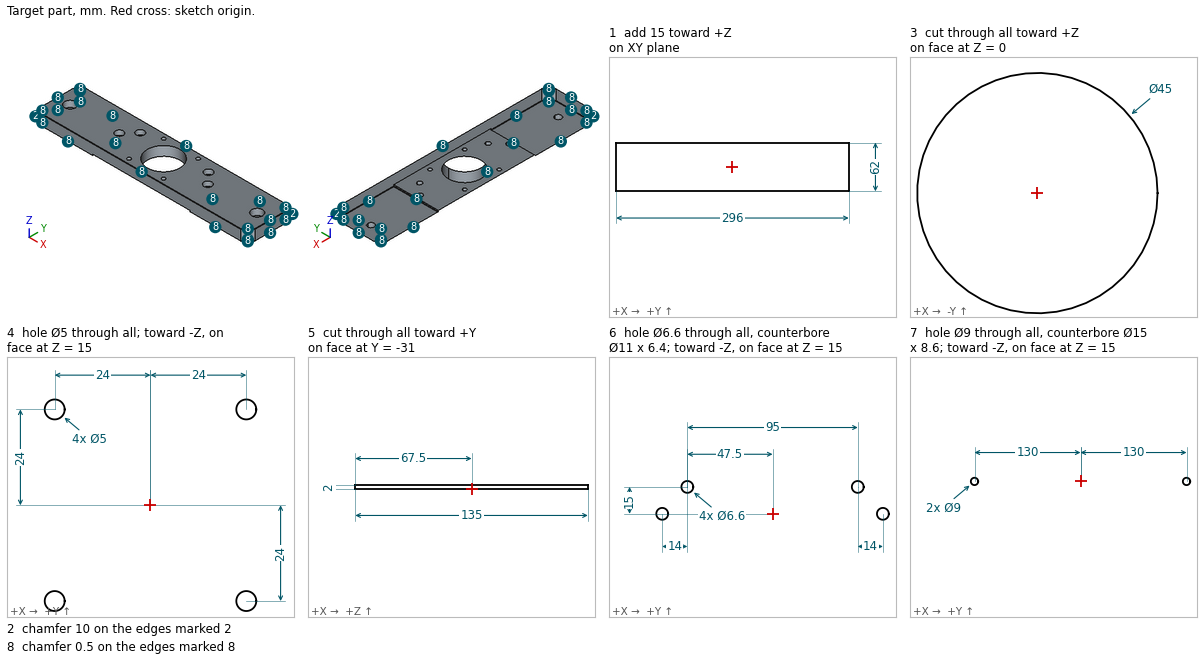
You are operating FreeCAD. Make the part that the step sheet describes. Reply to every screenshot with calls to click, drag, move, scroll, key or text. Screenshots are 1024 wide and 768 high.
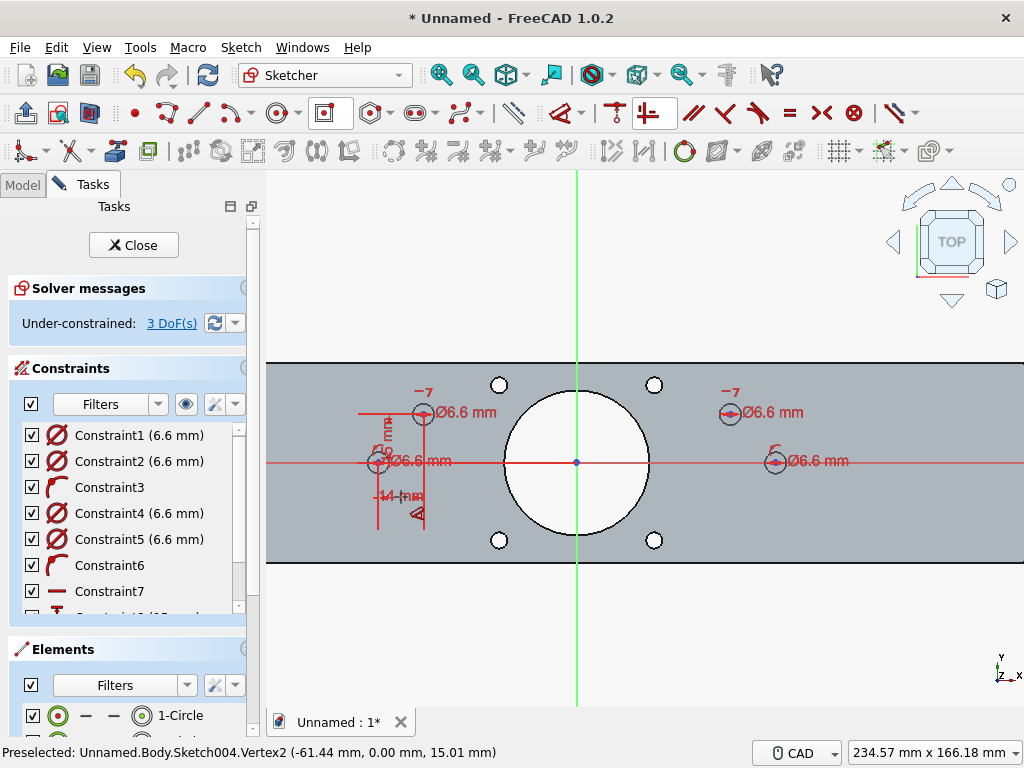
click(424, 414)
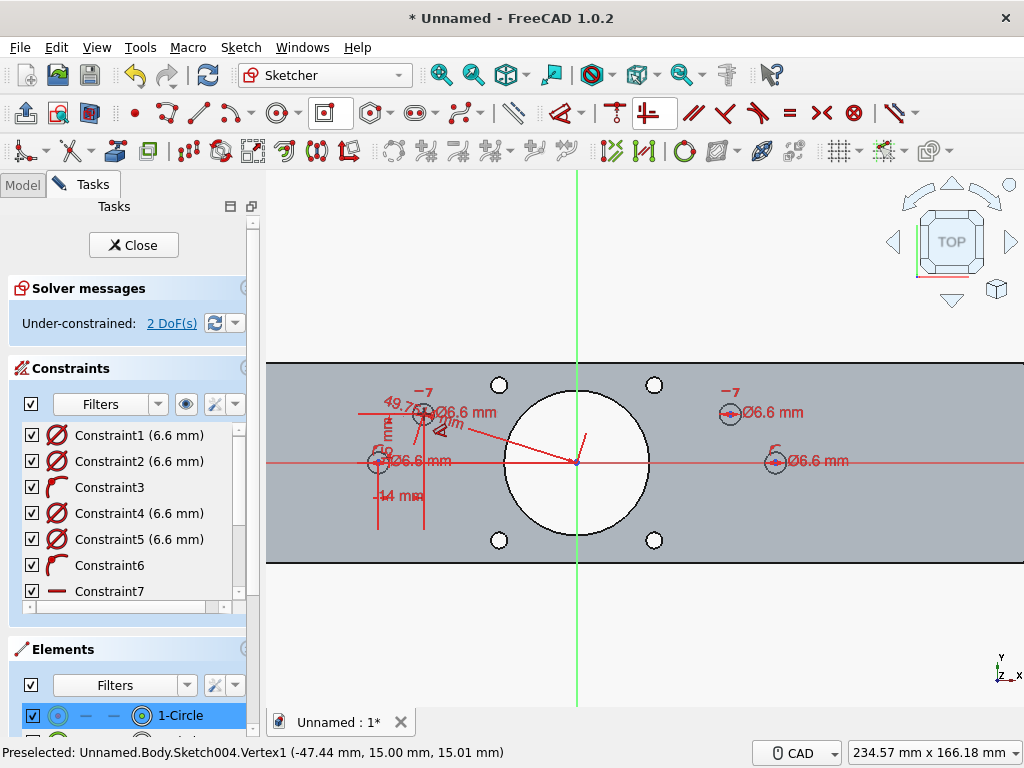
click(730, 414)
click(506, 380)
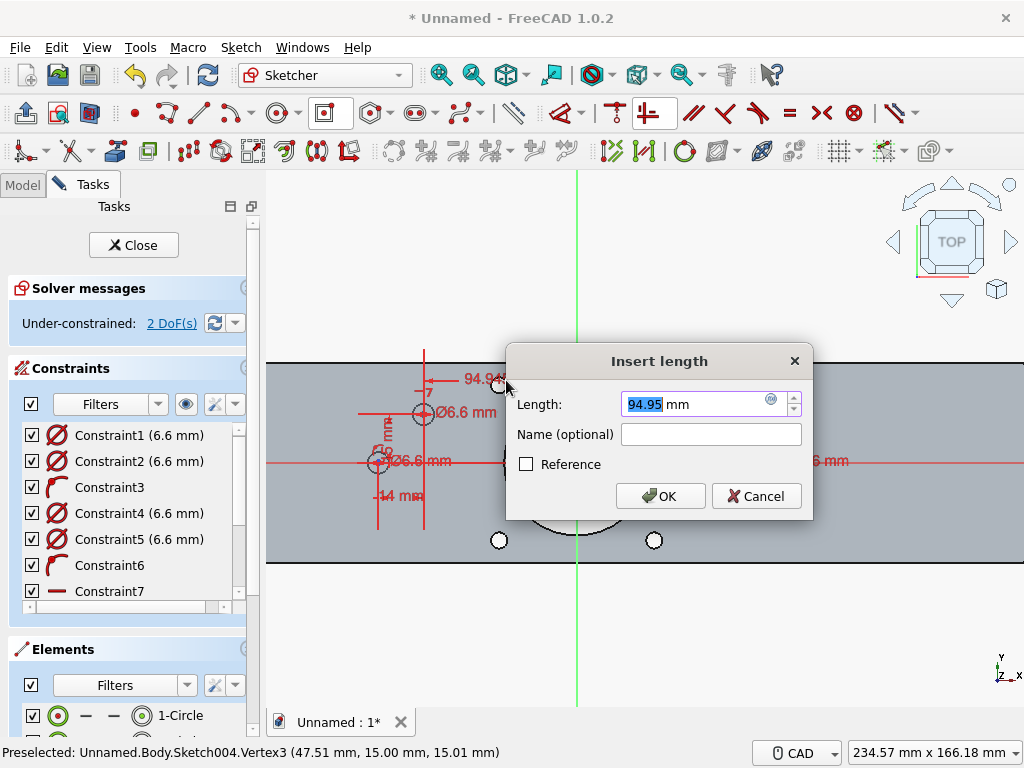
text(95)
key(Return)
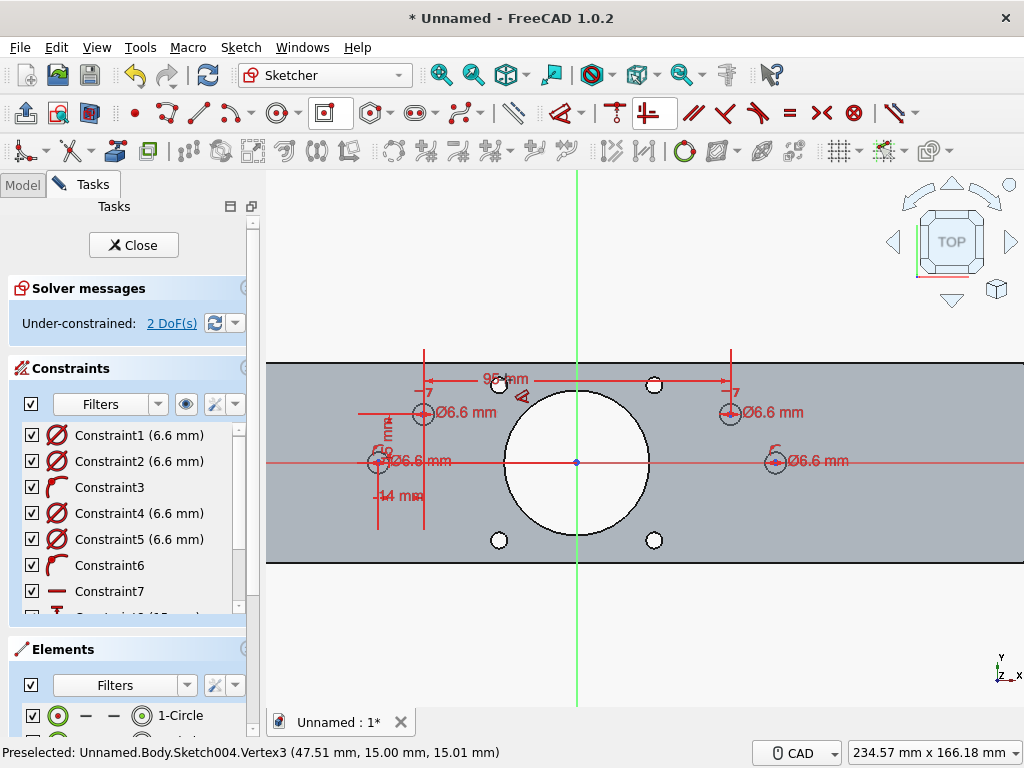
click(731, 414)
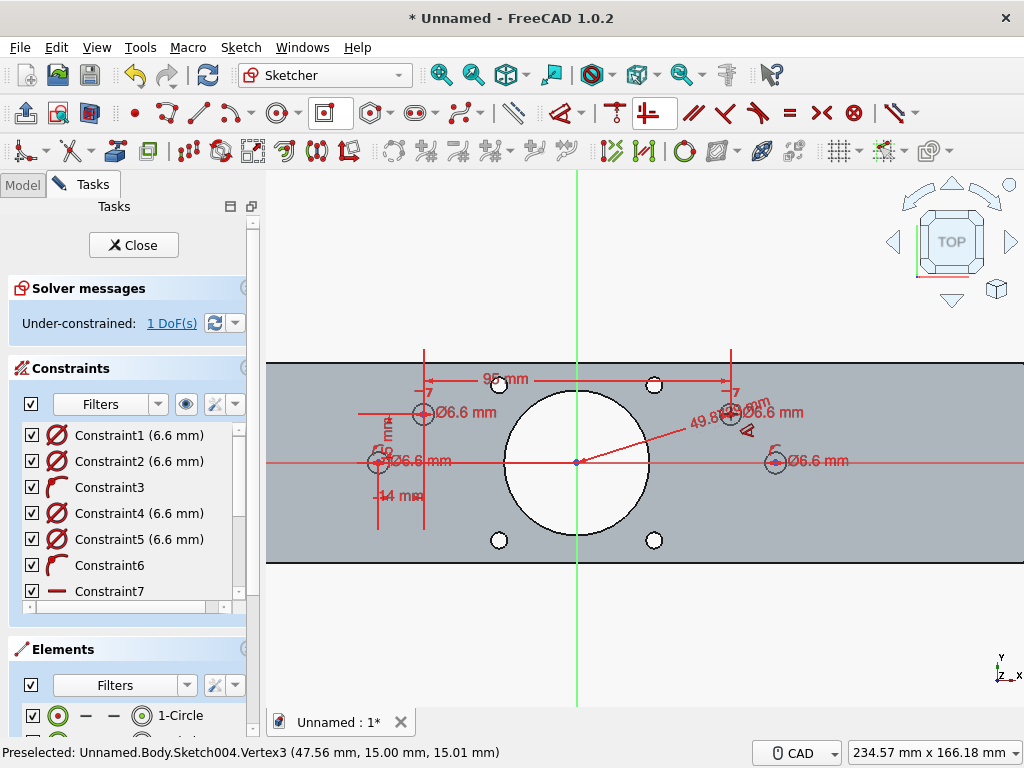
click(776, 463)
click(753, 497)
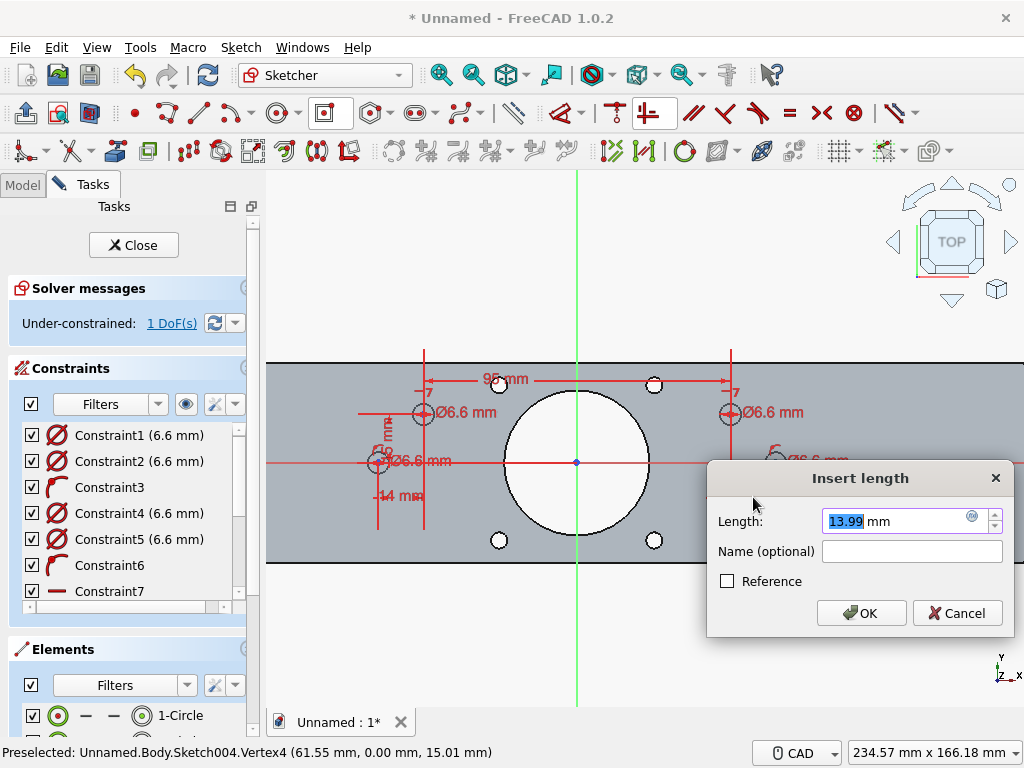
text(14)
key(Return)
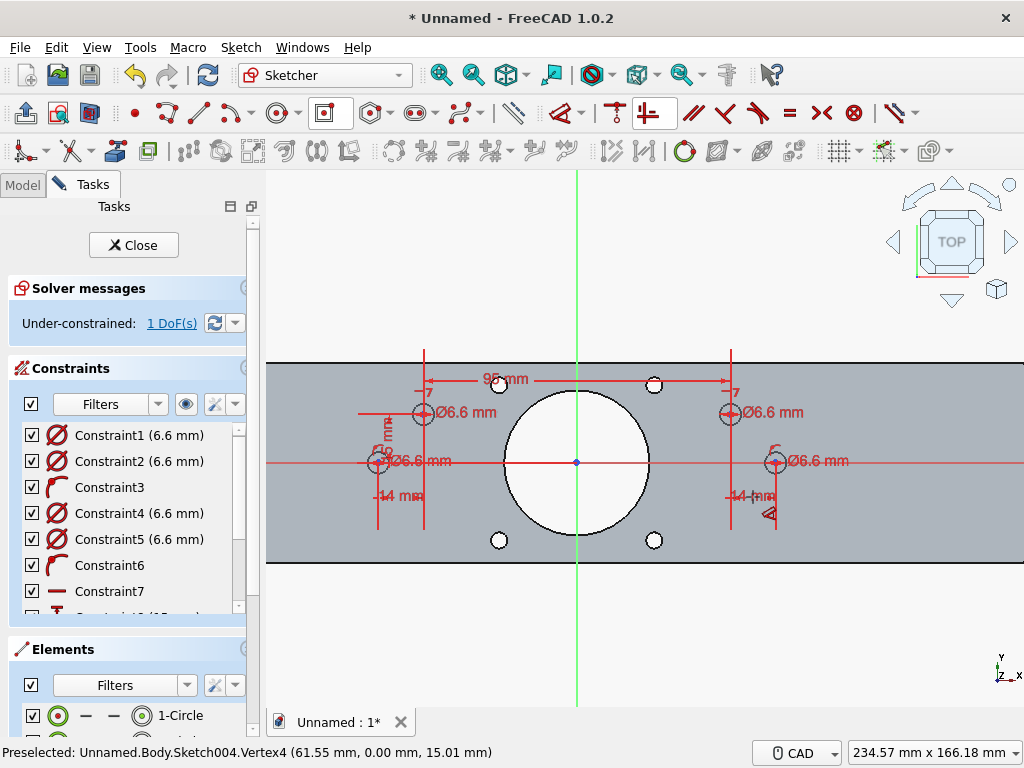
click(424, 414)
click(500, 497)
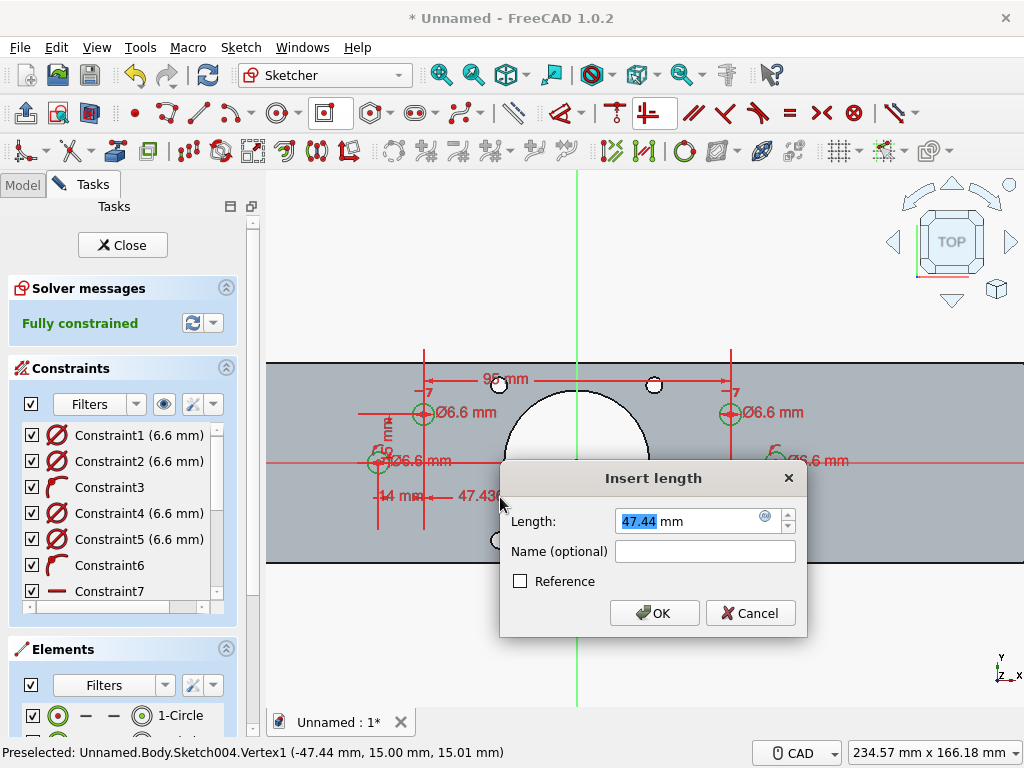
text(47.5)
key(Return)
key(Escape)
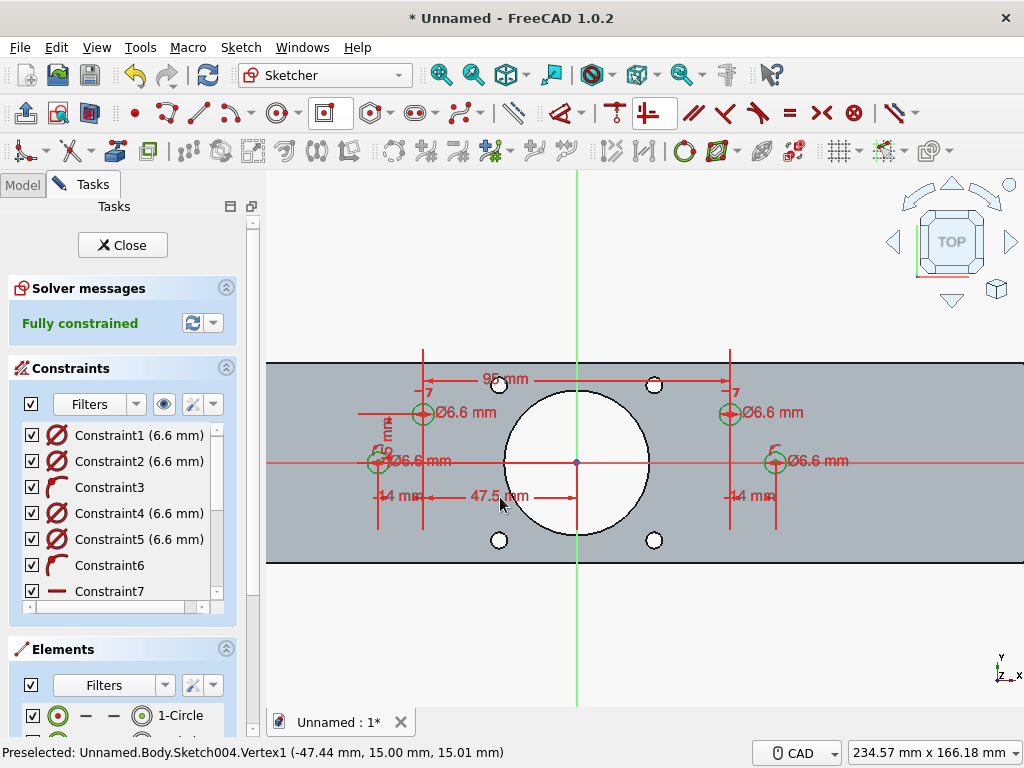
click(123, 245)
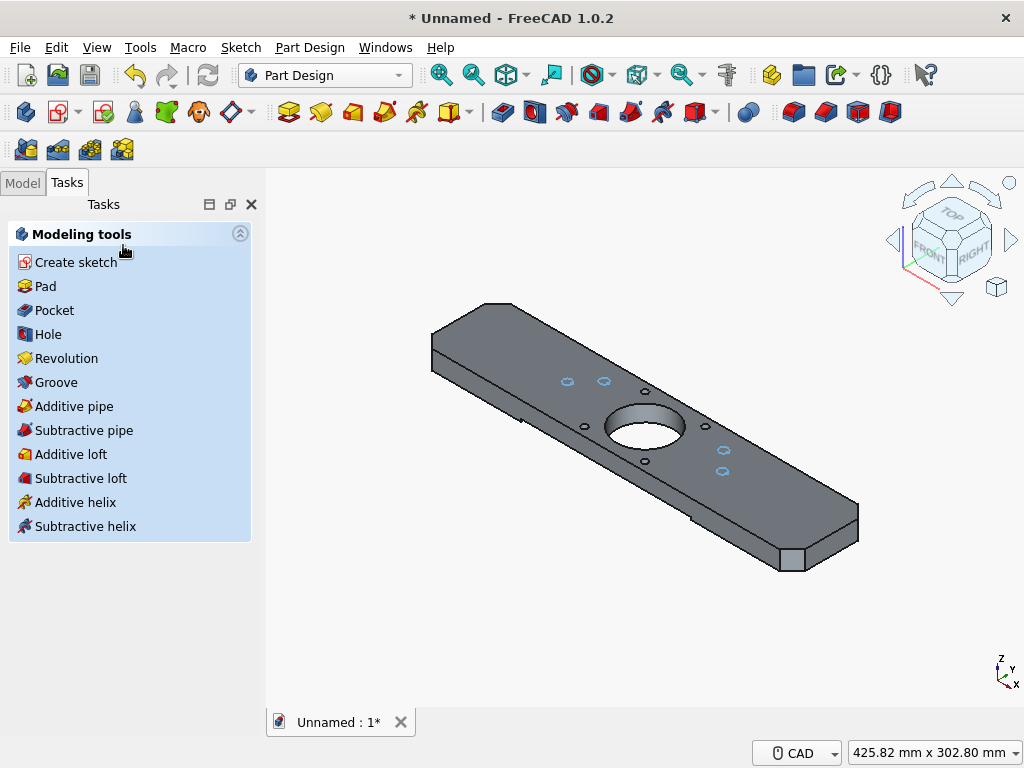
click(536, 112)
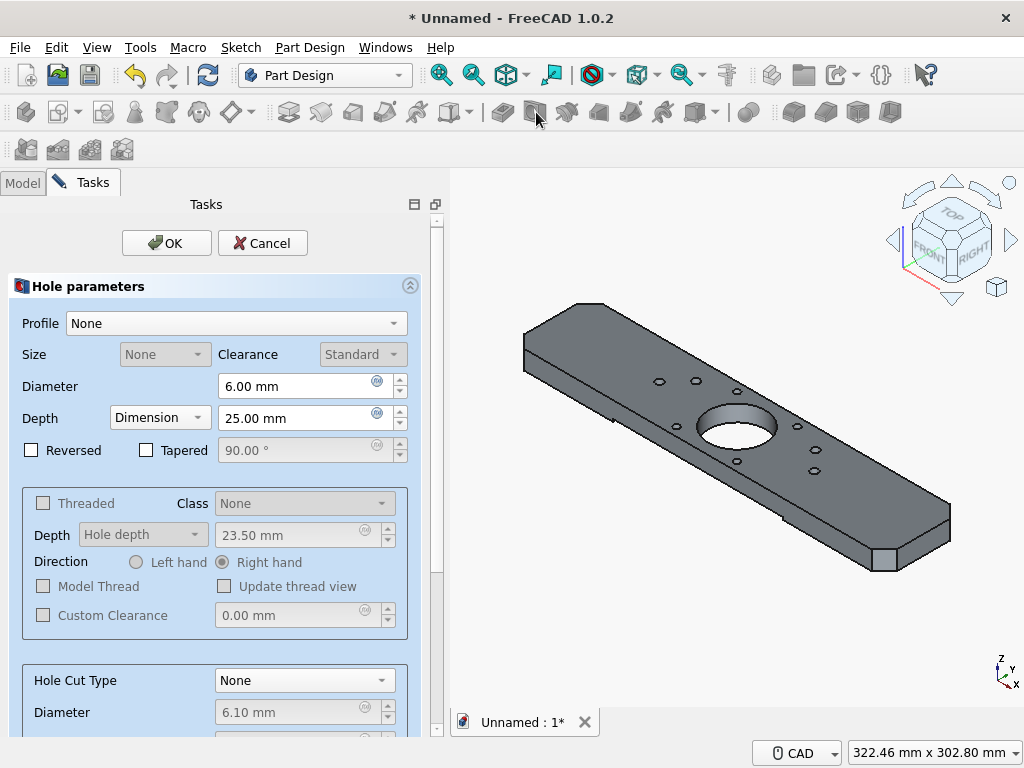
triple_click(305, 386)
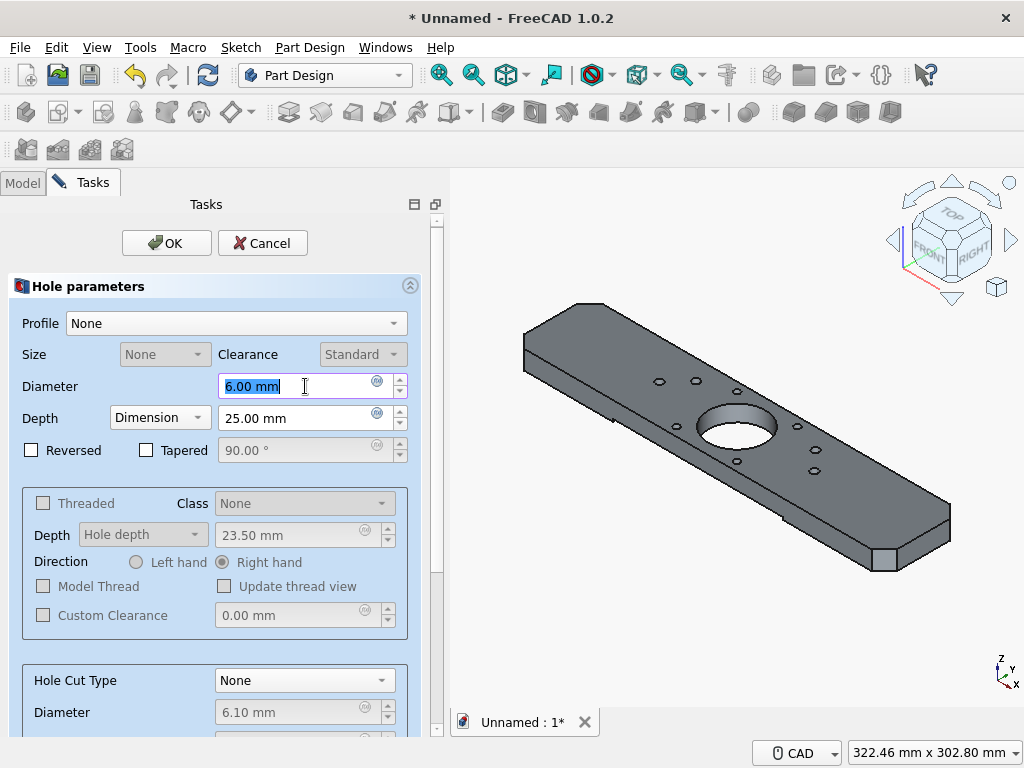
text(6.6)
key(Tab)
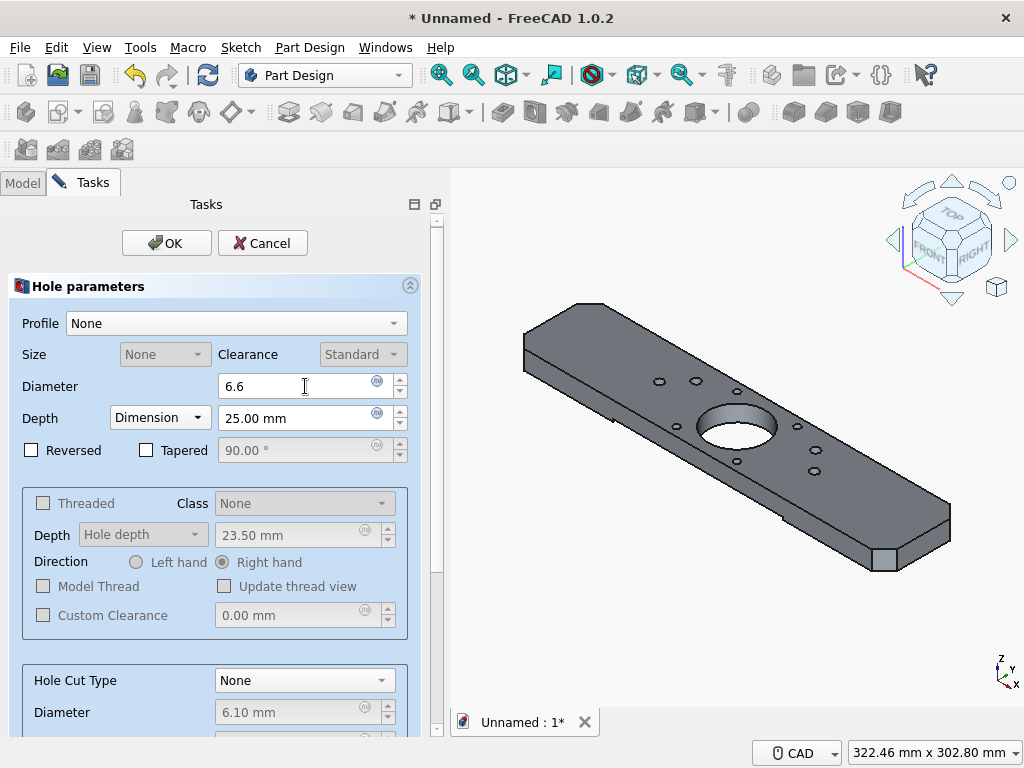
click(161, 418)